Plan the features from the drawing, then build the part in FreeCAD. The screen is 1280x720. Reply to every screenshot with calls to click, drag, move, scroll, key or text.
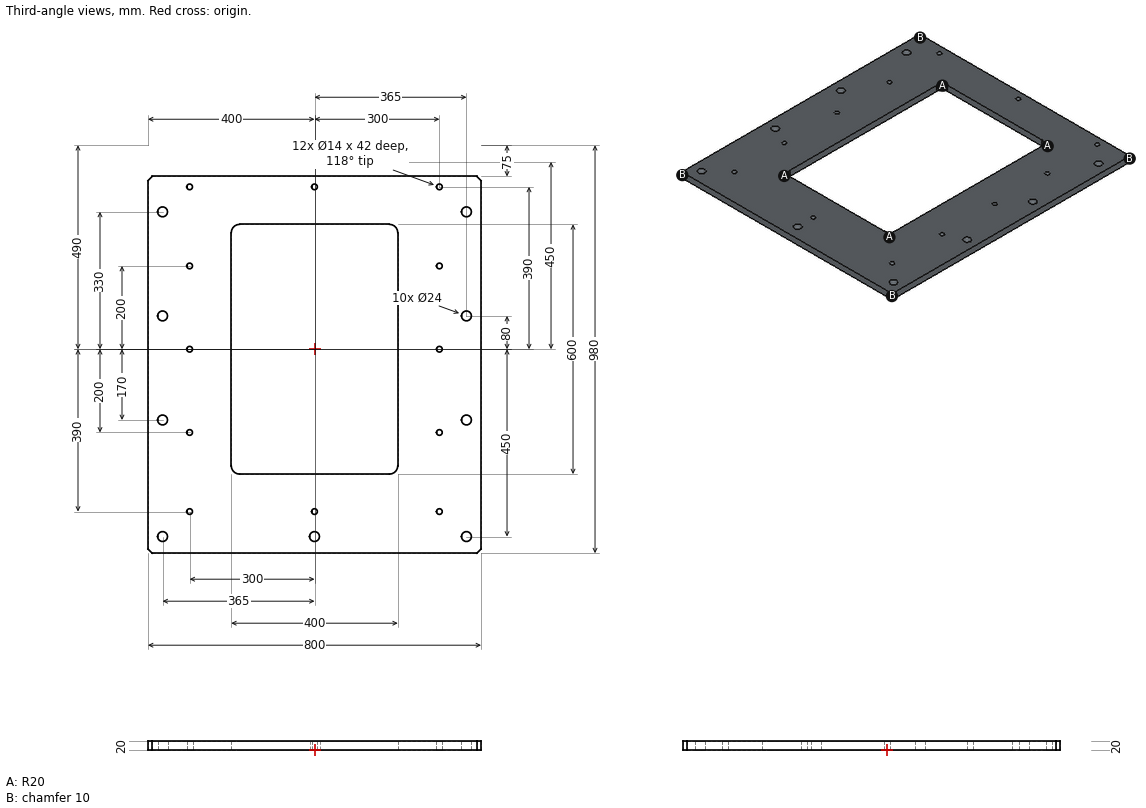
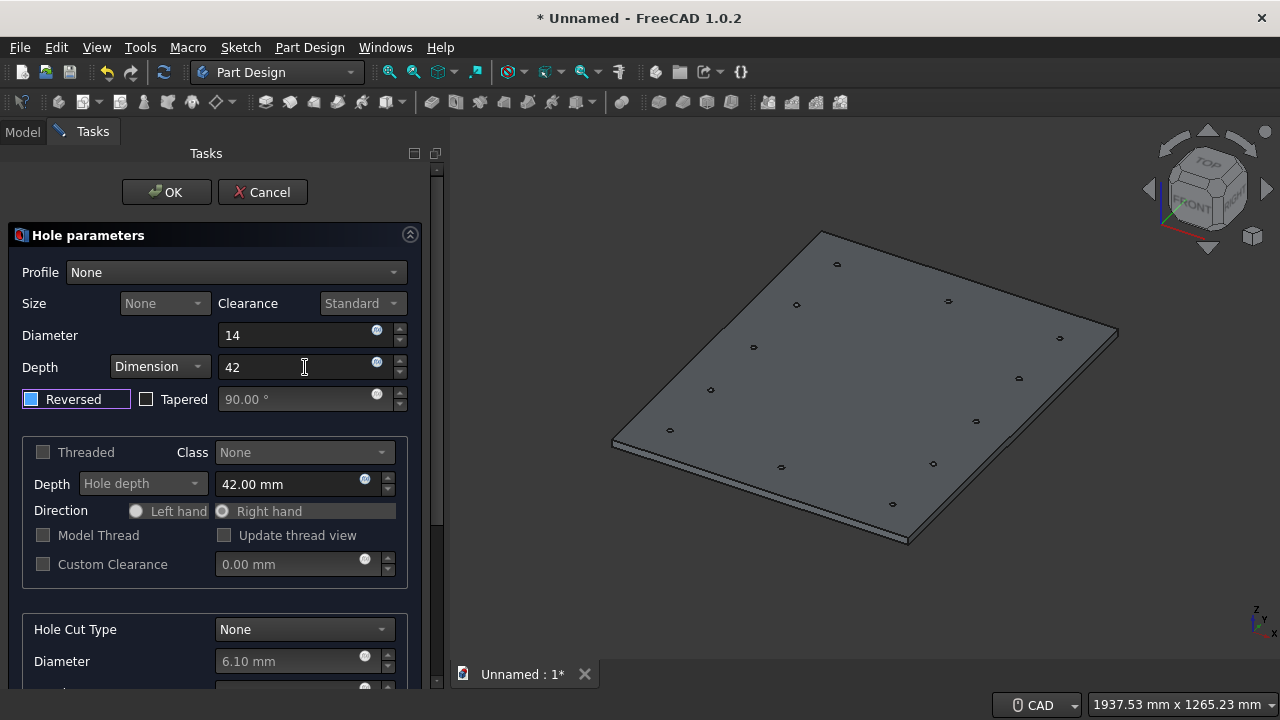
click(167, 192)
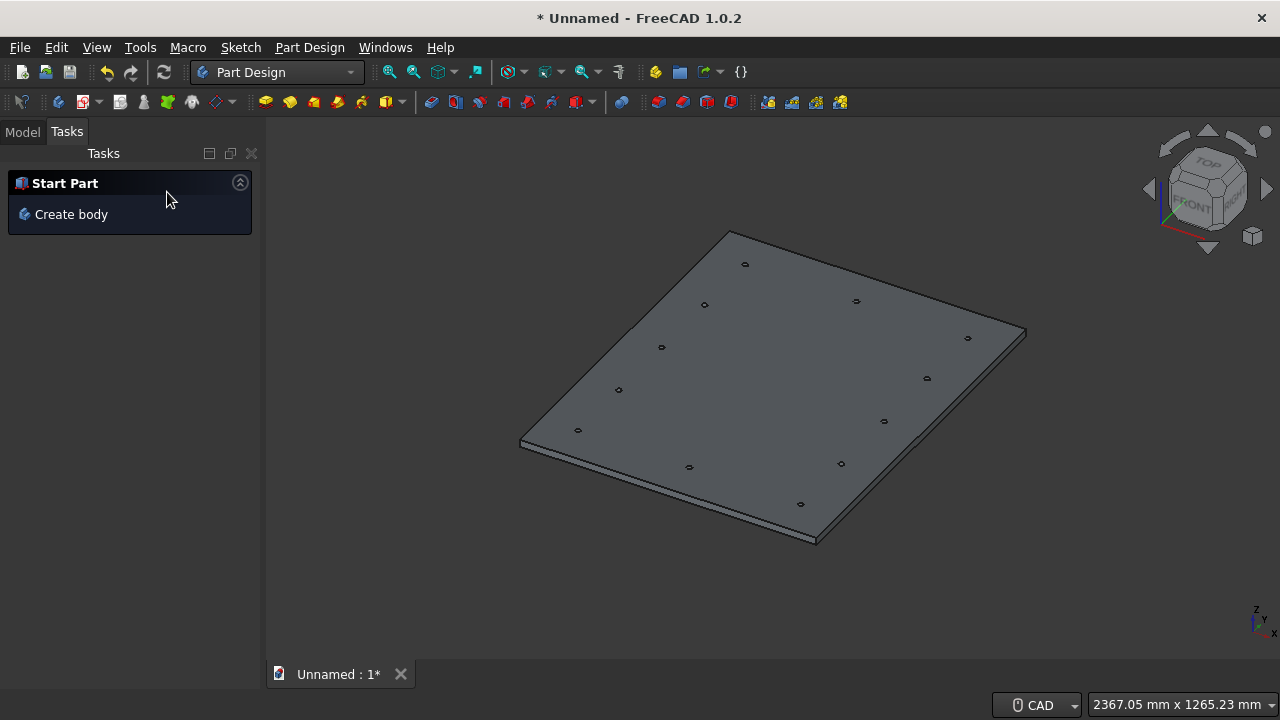
click(773, 383)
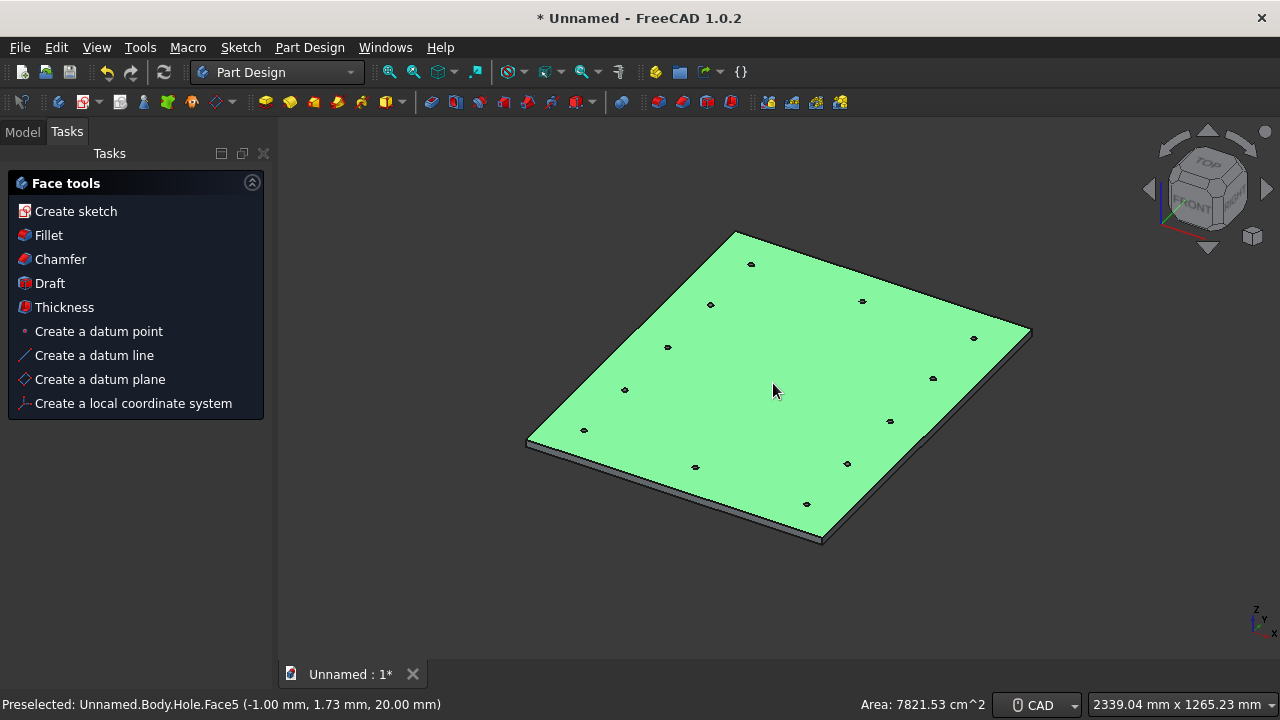
click(84, 102)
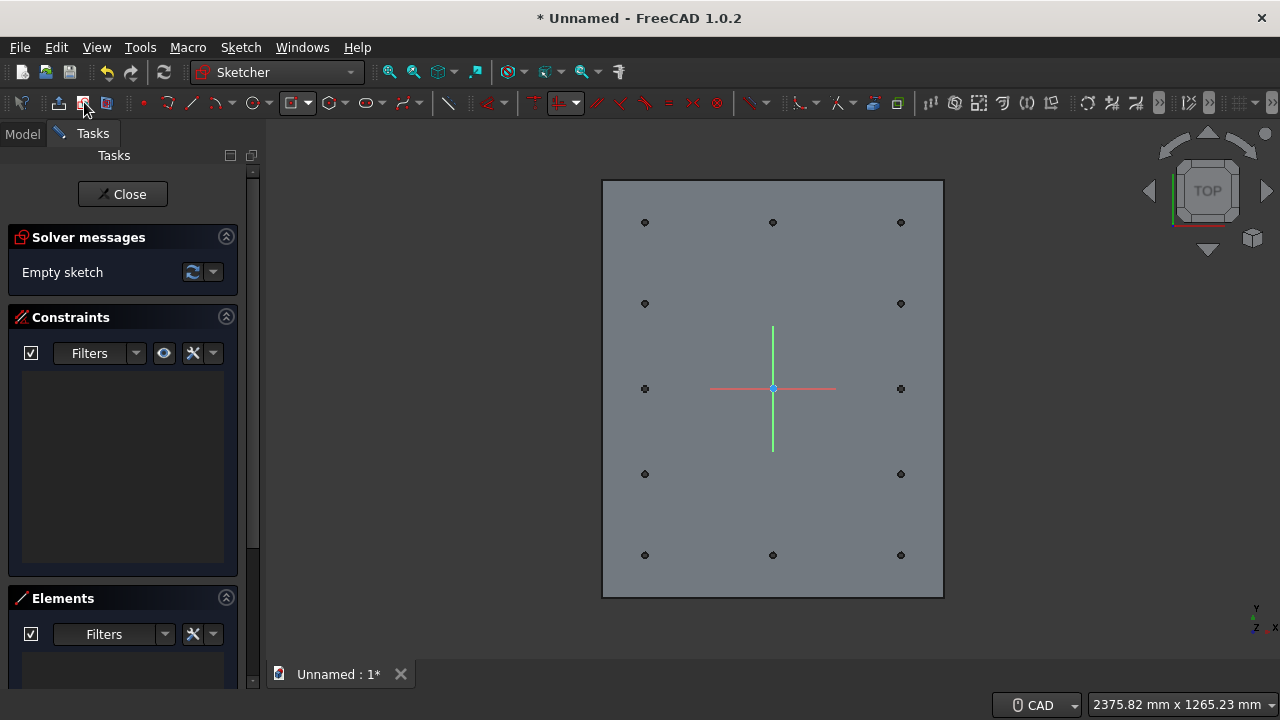
click(292, 104)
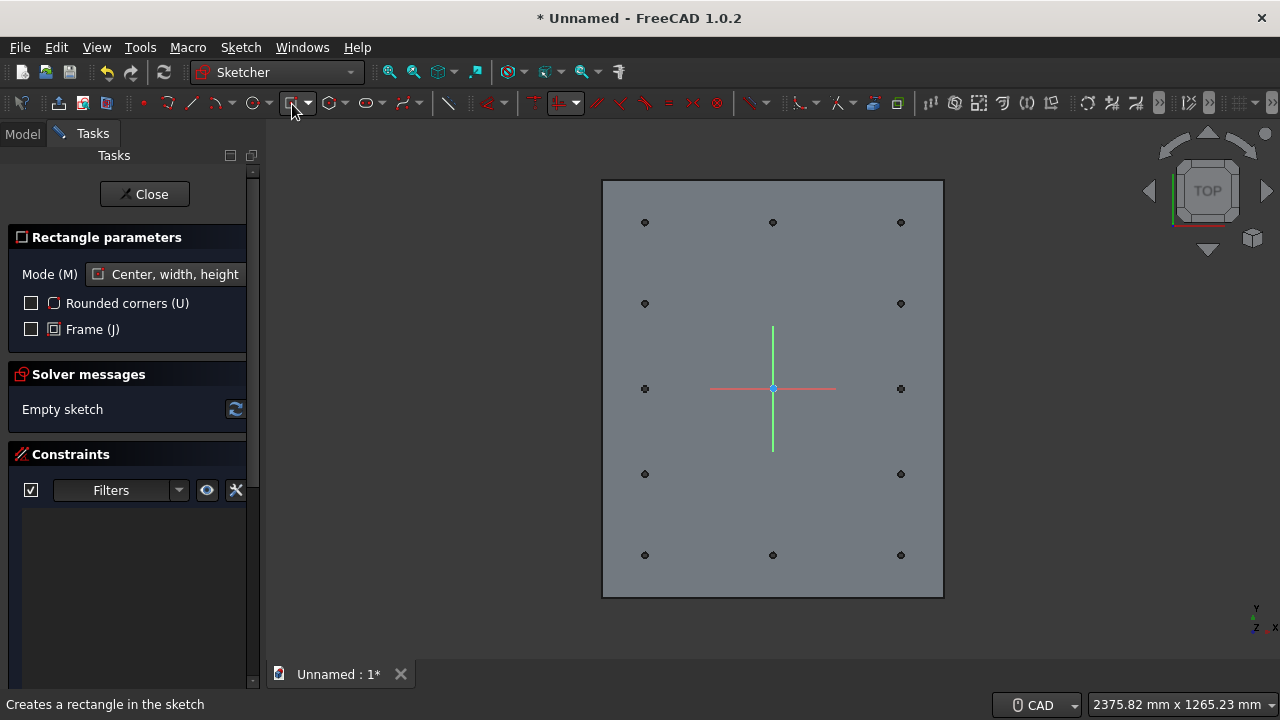
click(773, 389)
move(858, 261)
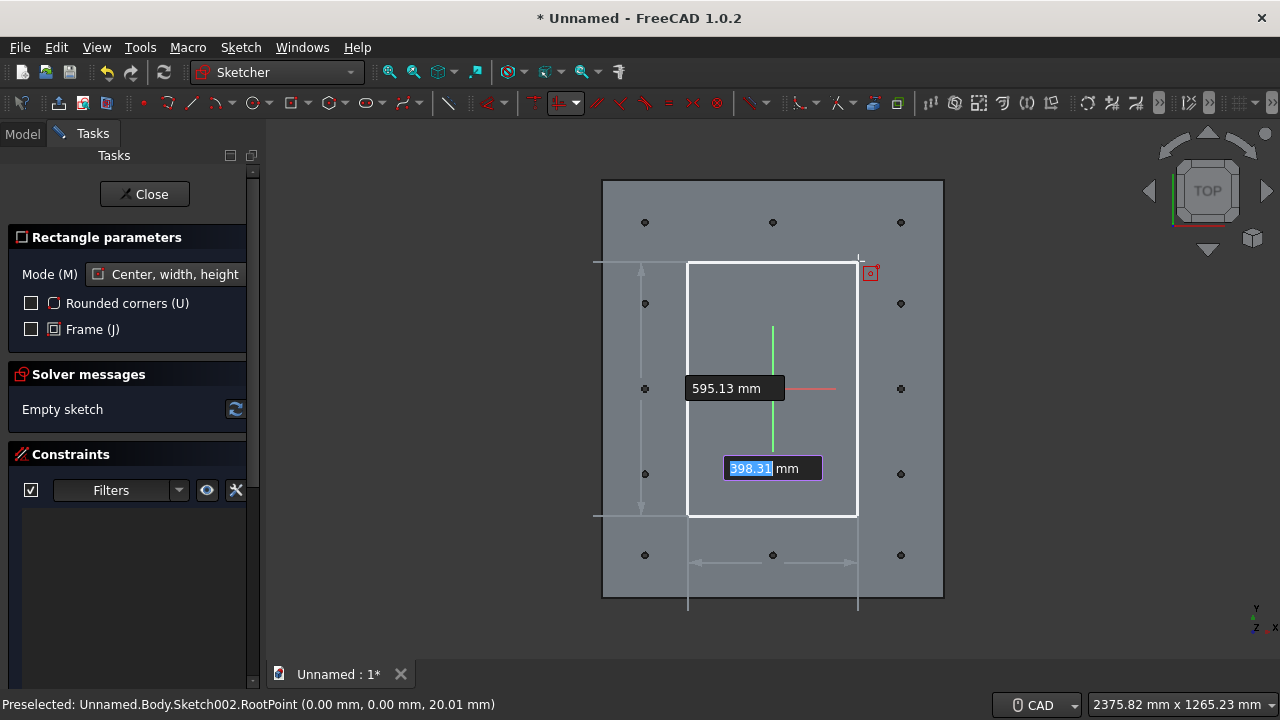
text(400)
key(Tab)
text(600)
key(Return)
key(Escape)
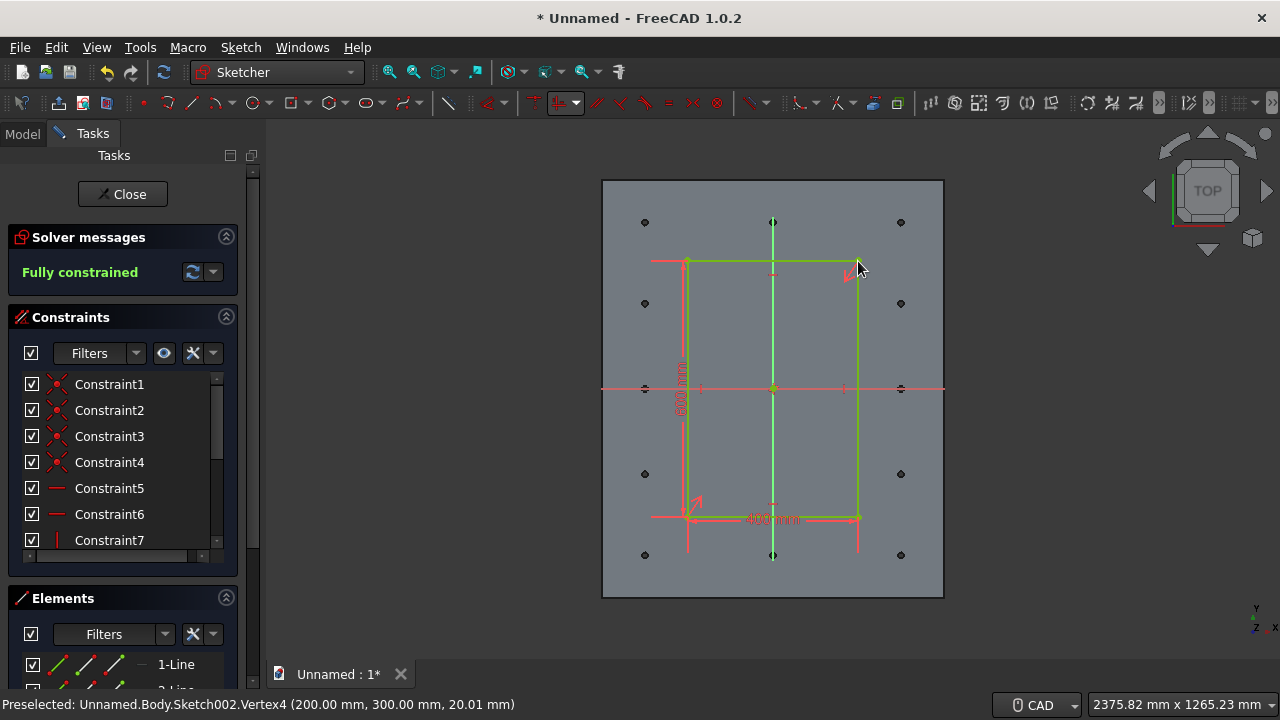
click(123, 194)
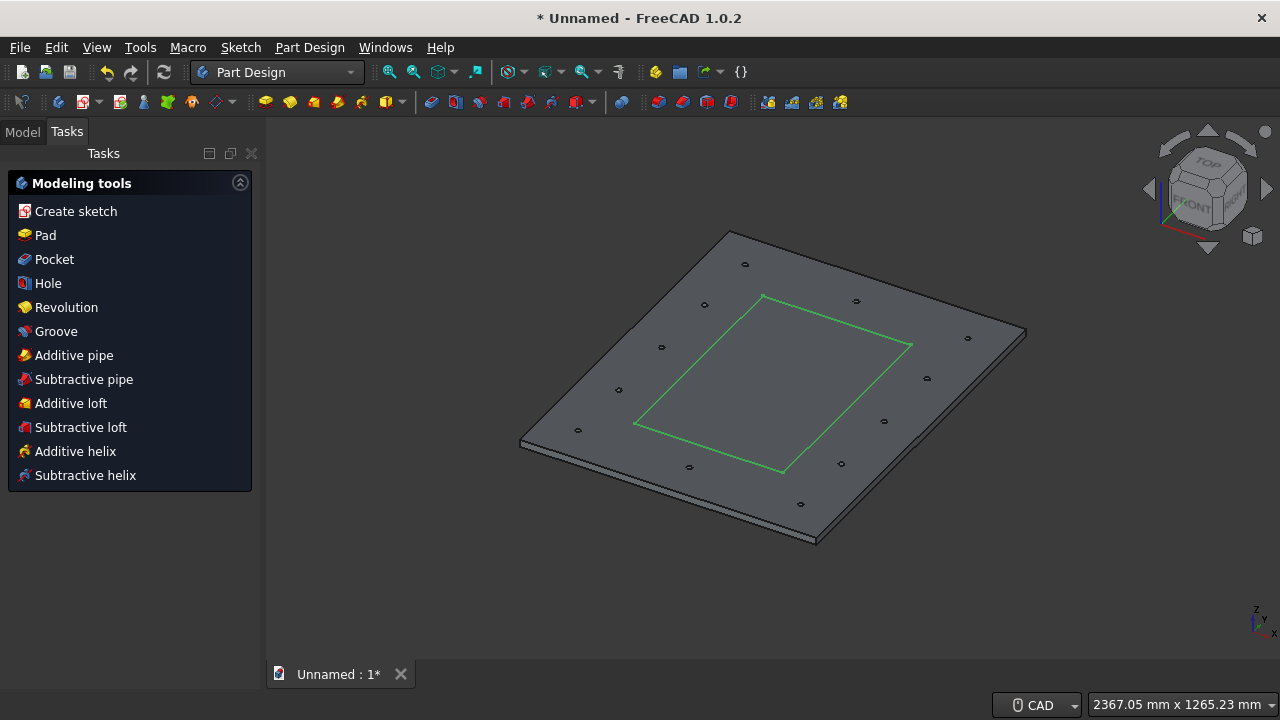
click(432, 102)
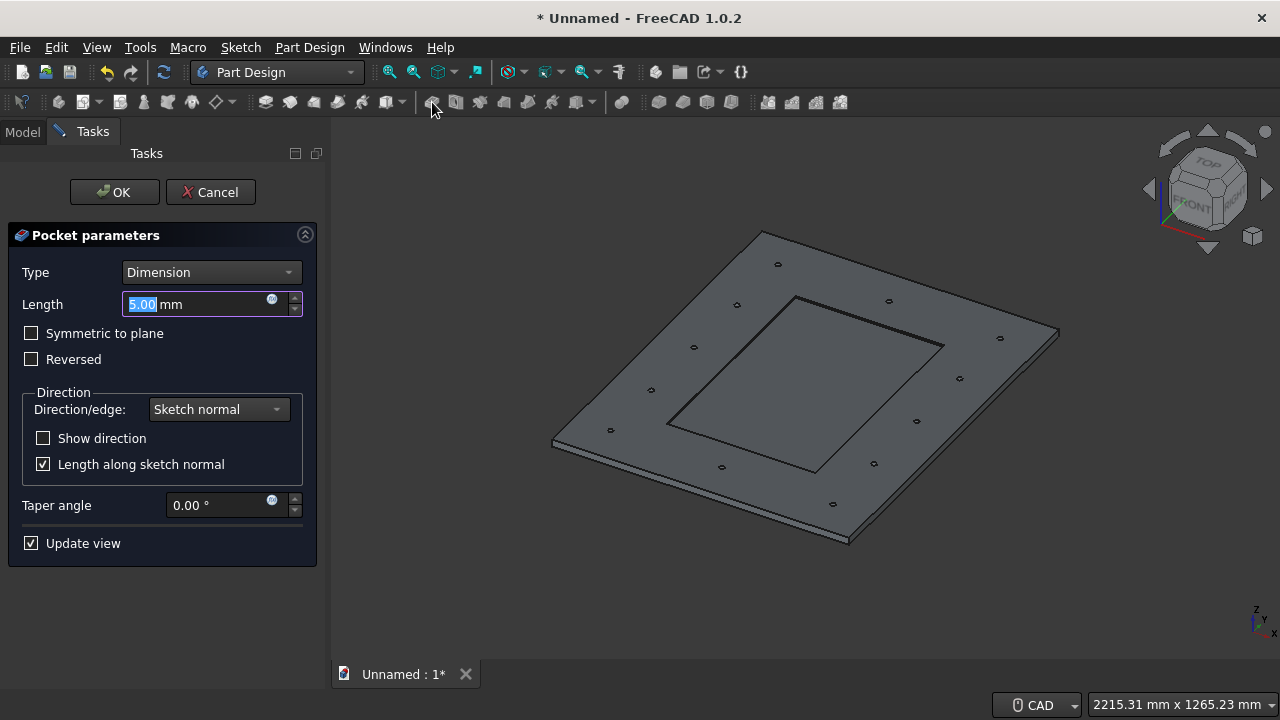
text(20)
key(Tab)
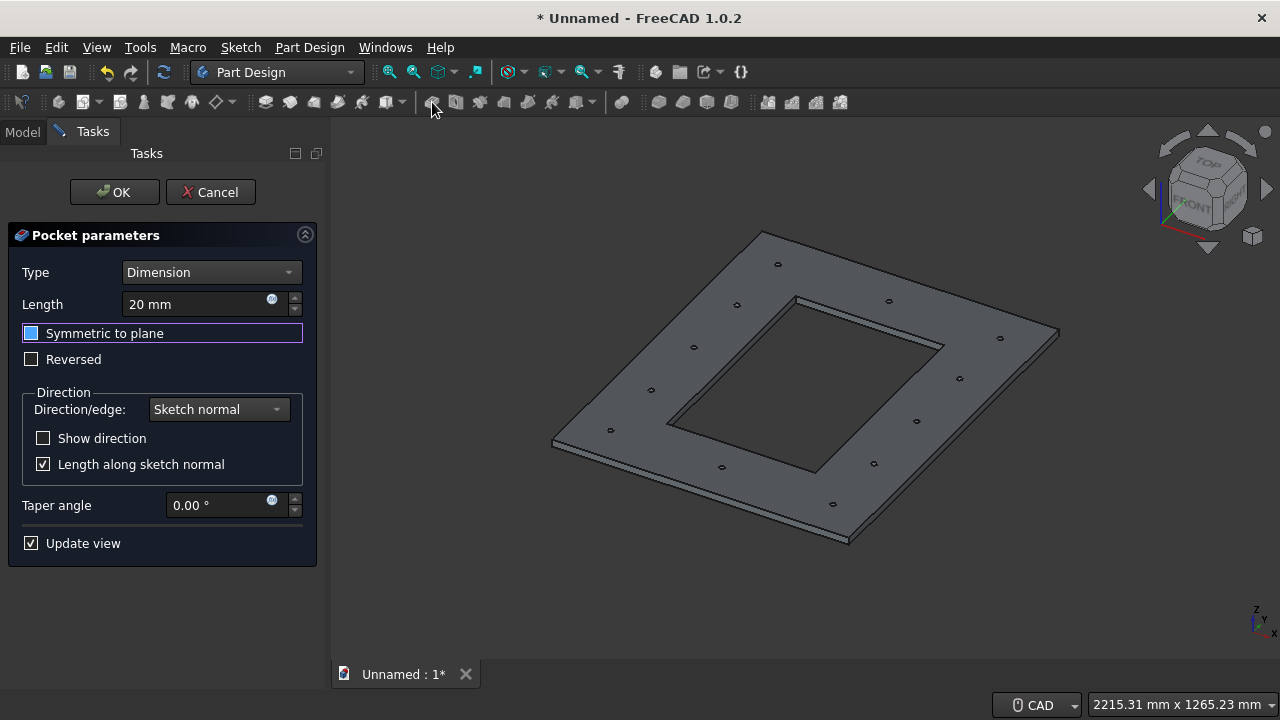
click(115, 192)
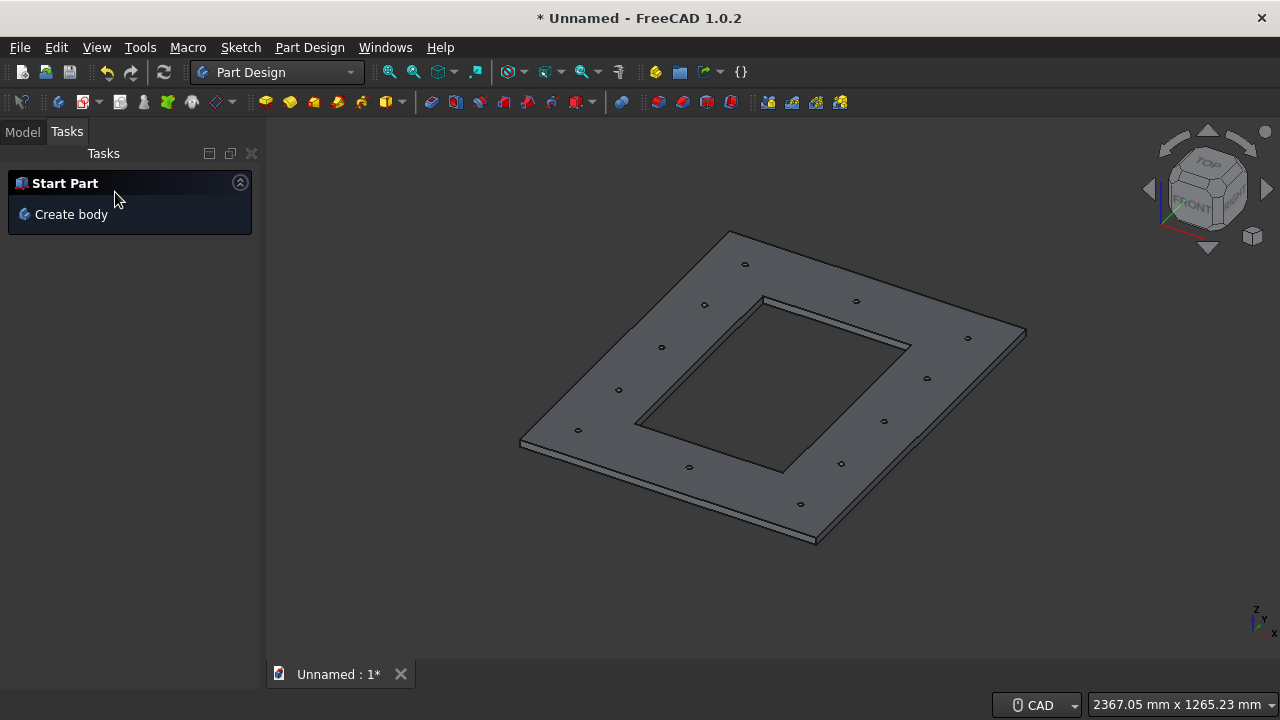
scroll(911, 348, up, 8)